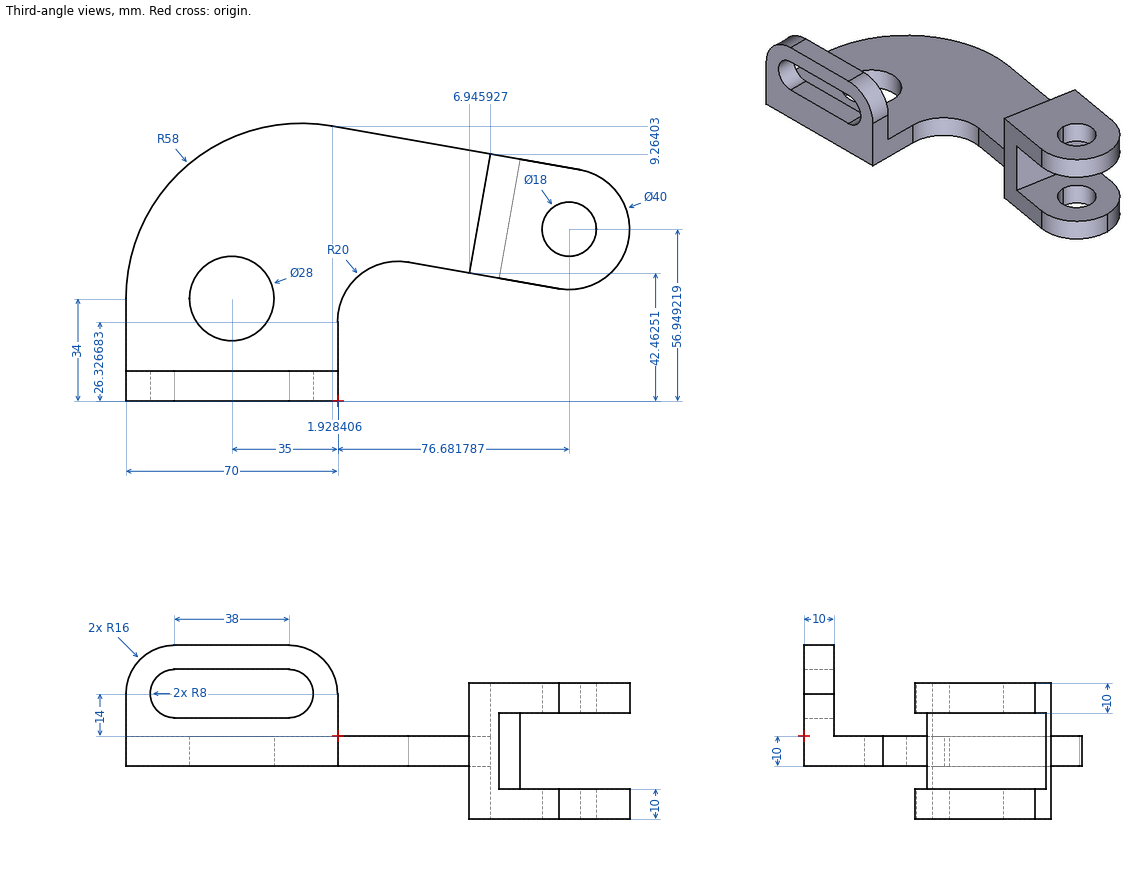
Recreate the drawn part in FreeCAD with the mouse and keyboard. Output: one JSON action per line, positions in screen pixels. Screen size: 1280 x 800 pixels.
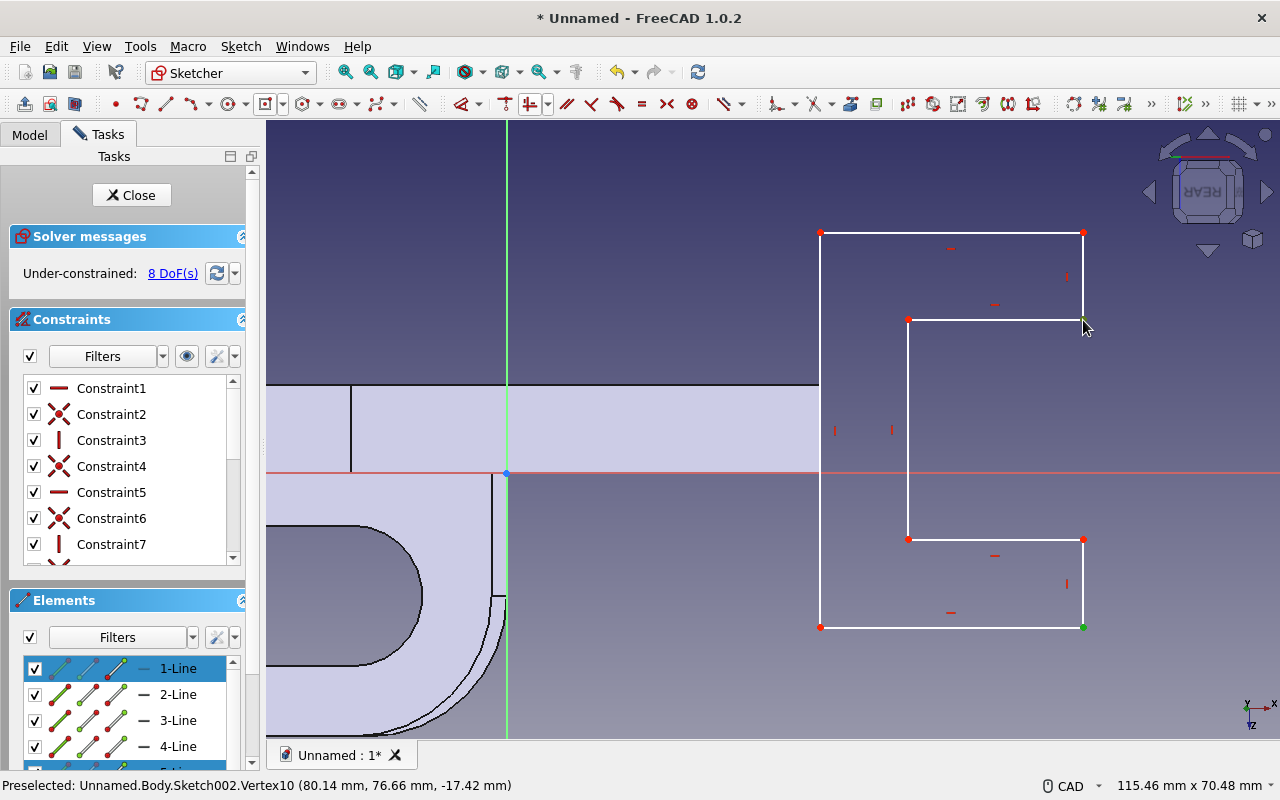
{"action": "left_click", "coordinate": [353, 473]}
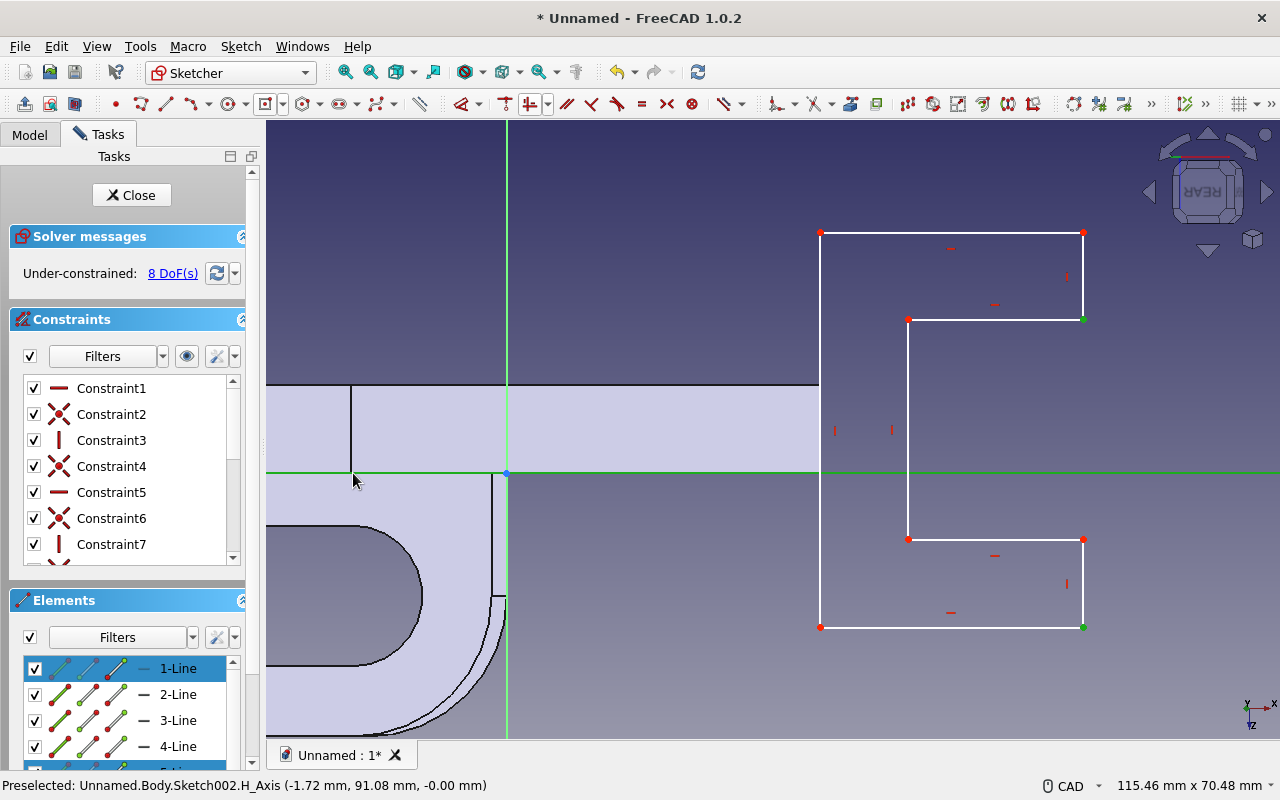
{"action": "left_click", "coordinate": [667, 104]}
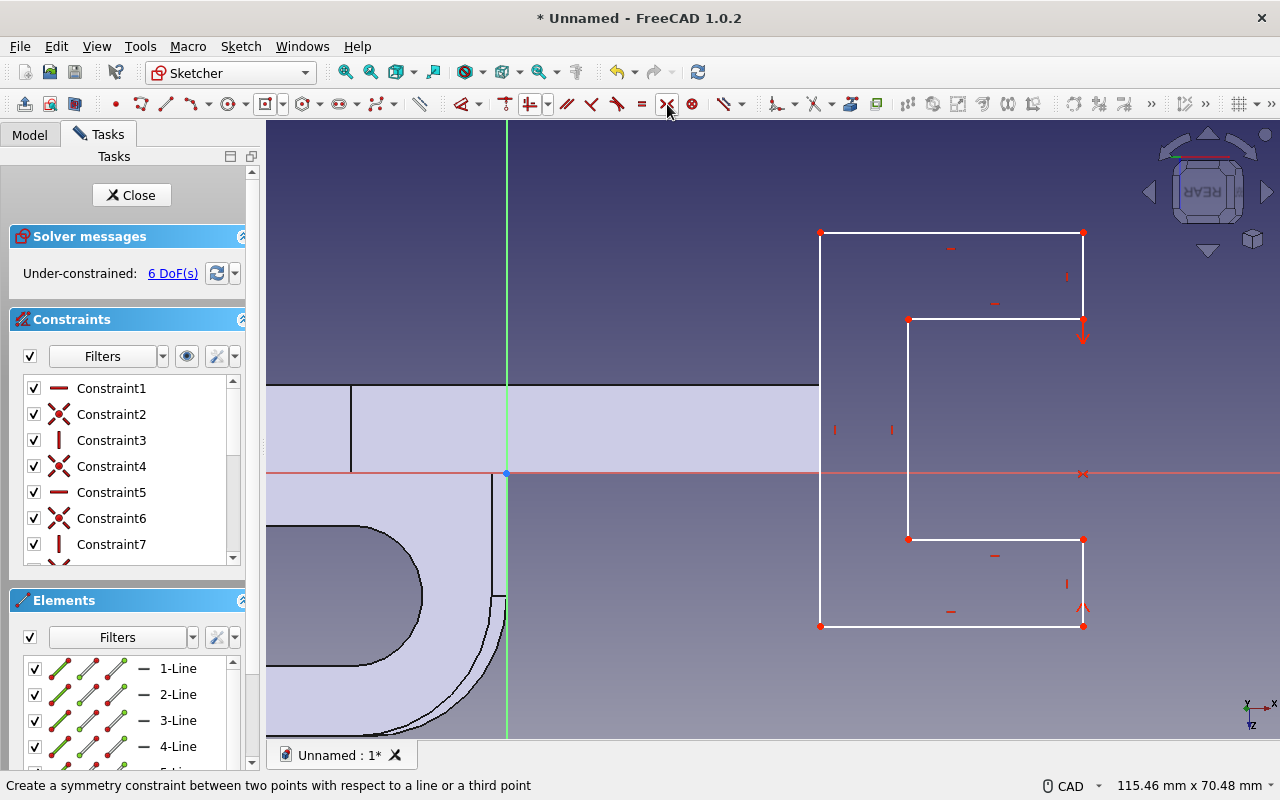
{"action": "key", "text": "d"}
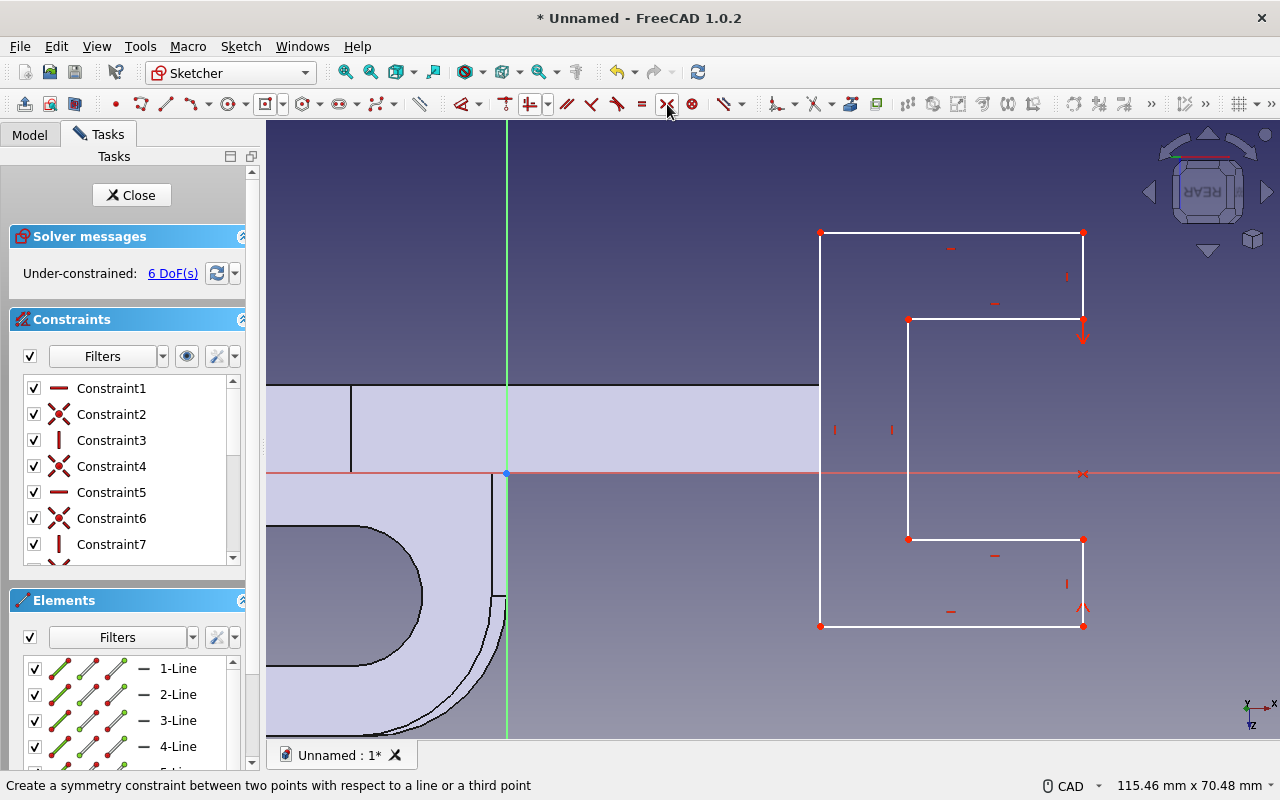
{"action": "left_click", "coordinate": [899, 627]}
{"action": "left_click", "coordinate": [952, 661]}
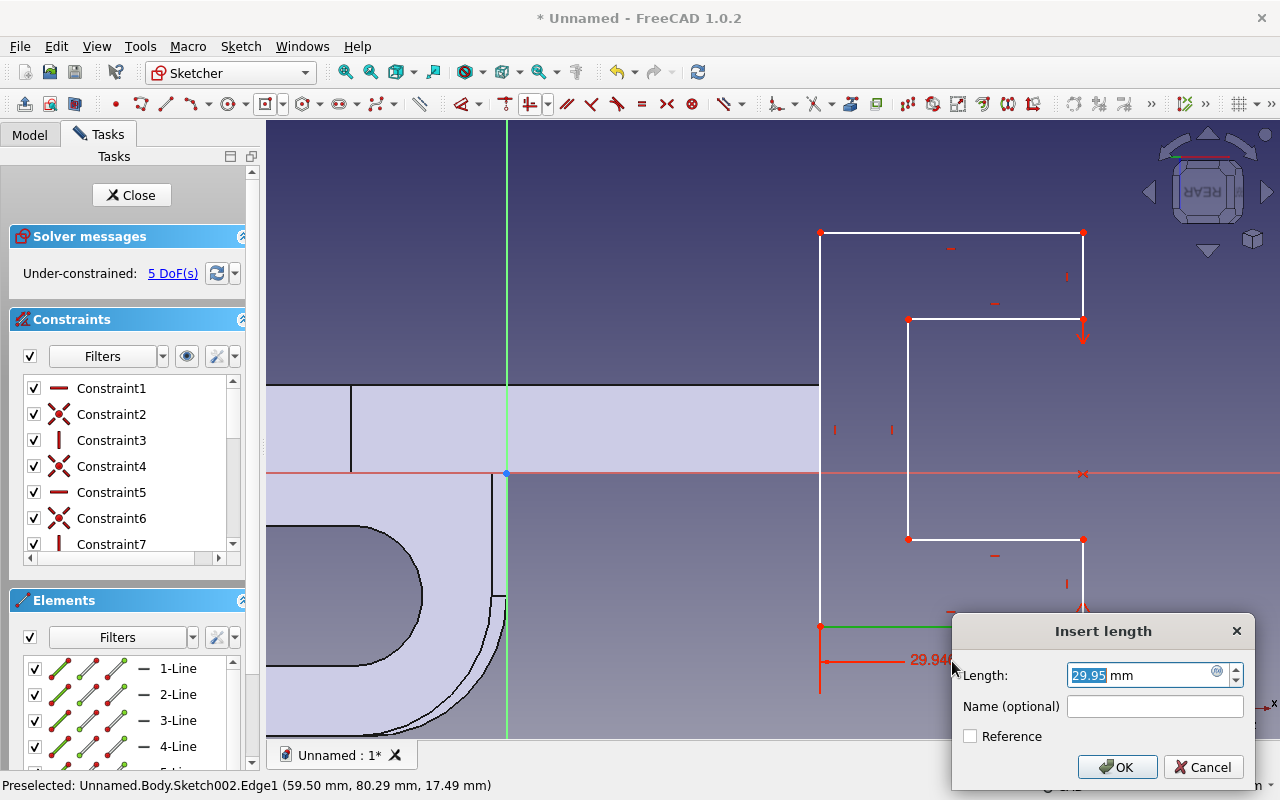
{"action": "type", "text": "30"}
{"action": "key", "text": "Return"}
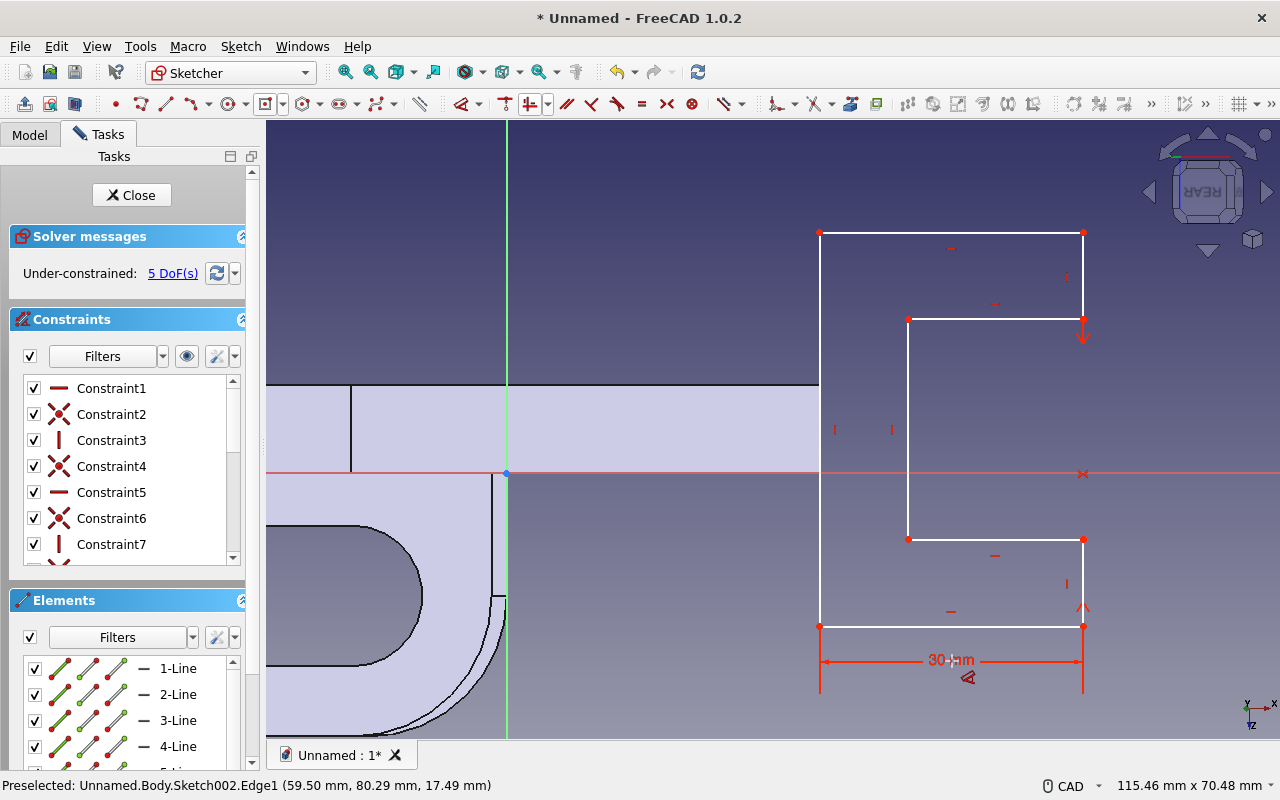
{"action": "left_click", "coordinate": [1083, 601]}
{"action": "left_click", "coordinate": [1049, 583]}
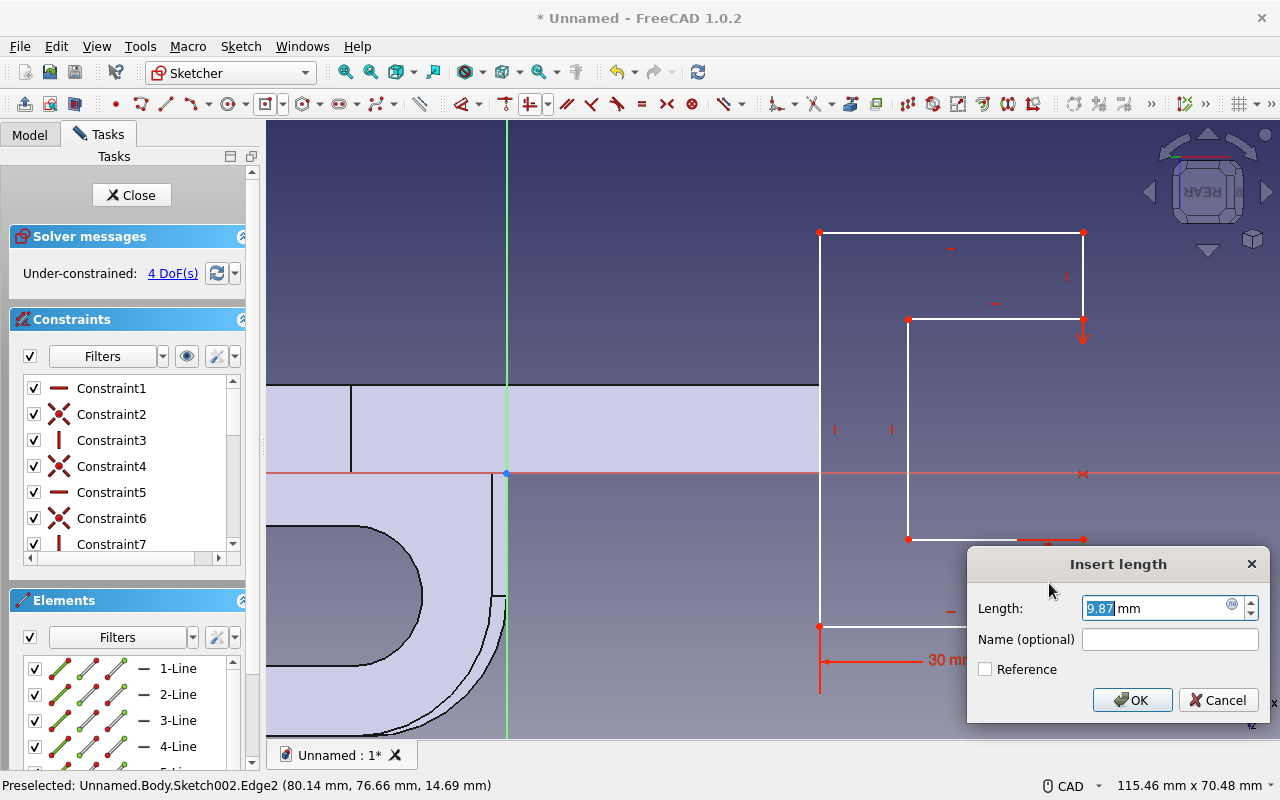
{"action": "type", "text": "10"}
{"action": "key", "text": "Return"}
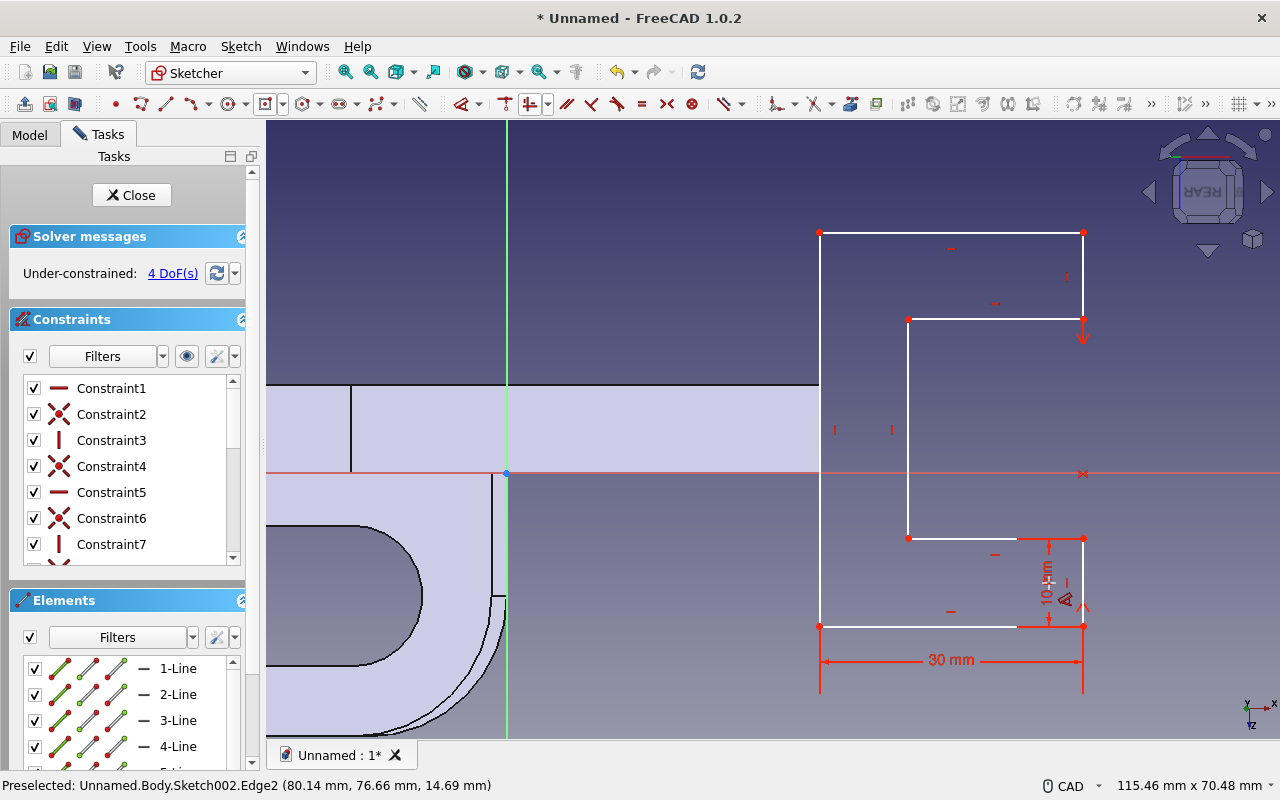
{"action": "left_click", "coordinate": [1031, 539]}
{"action": "left_click", "coordinate": [955, 573]}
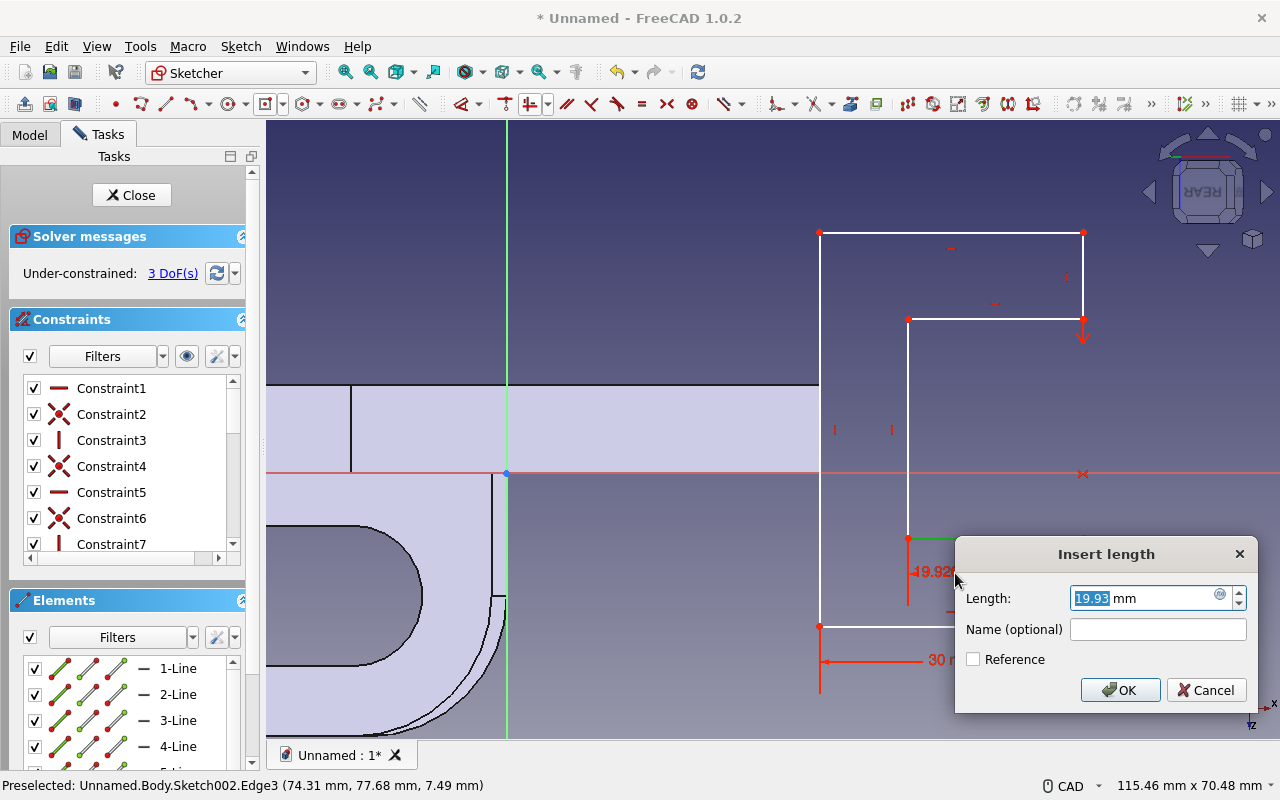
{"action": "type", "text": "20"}
{"action": "key", "text": "Return"}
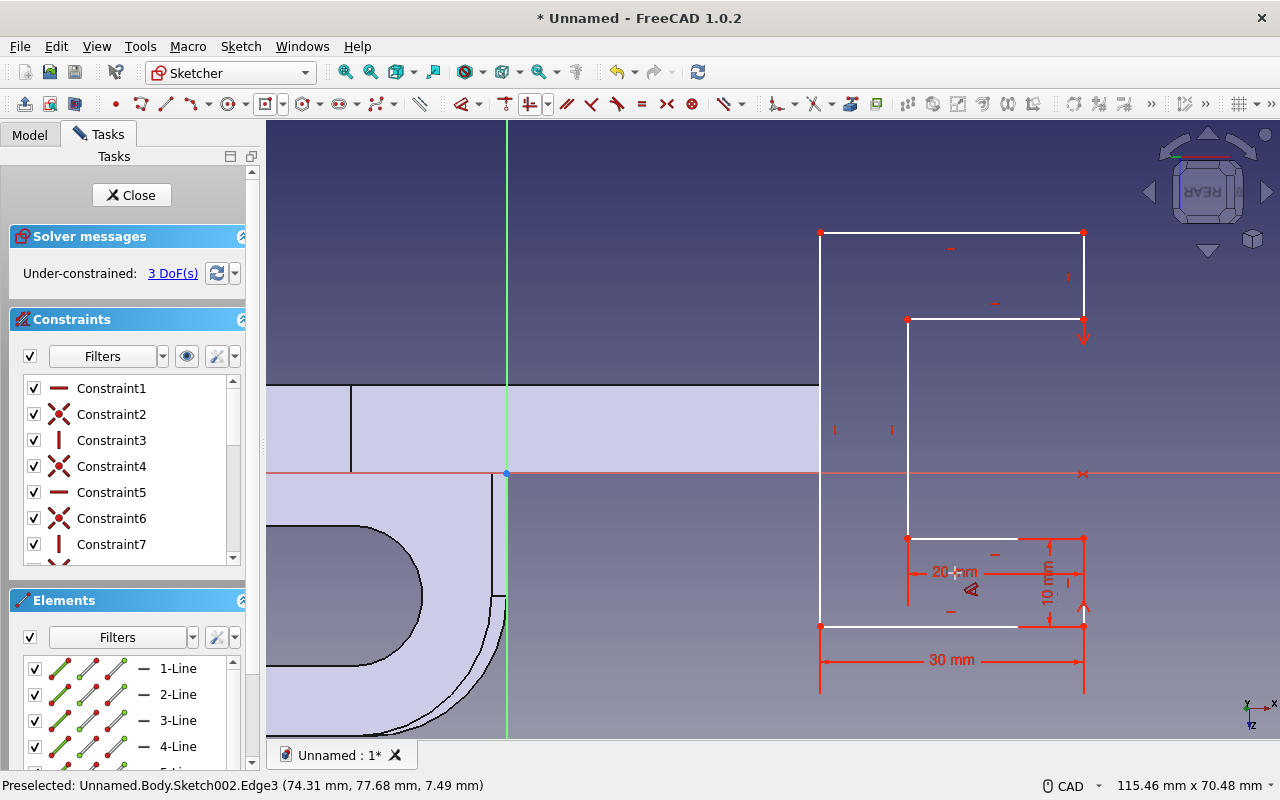
{"action": "left_click", "coordinate": [908, 473]}
{"action": "left_click", "coordinate": [942, 429]}